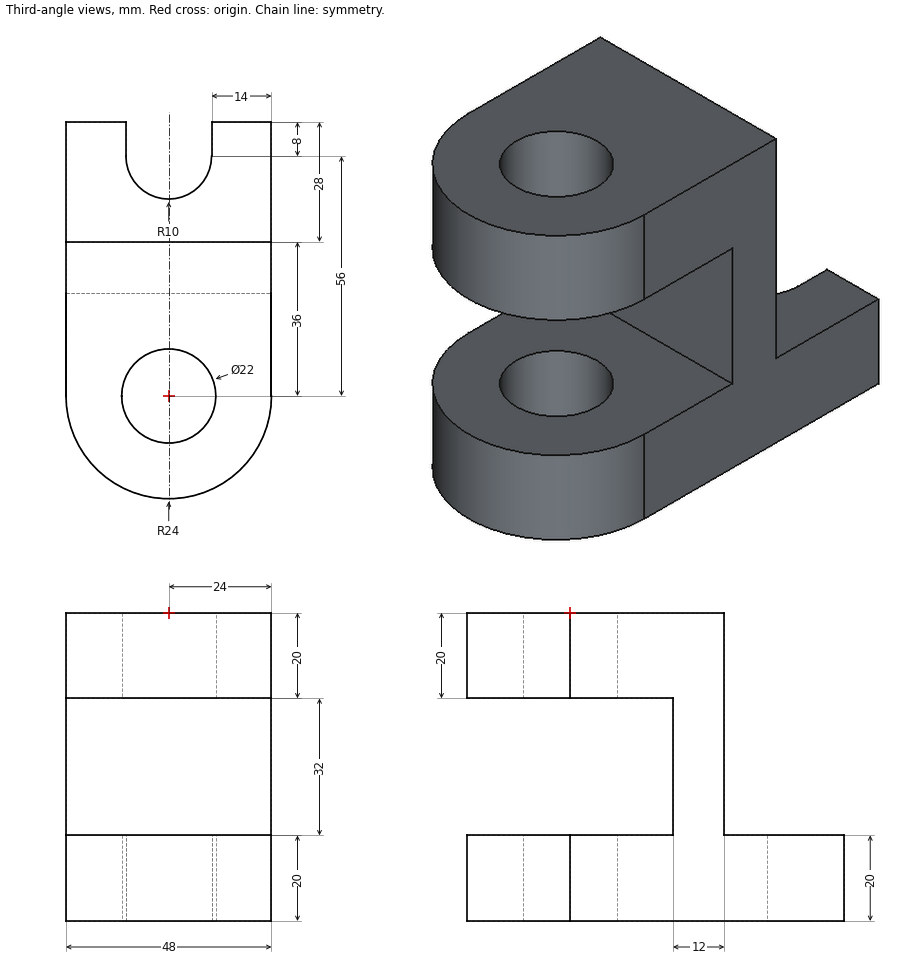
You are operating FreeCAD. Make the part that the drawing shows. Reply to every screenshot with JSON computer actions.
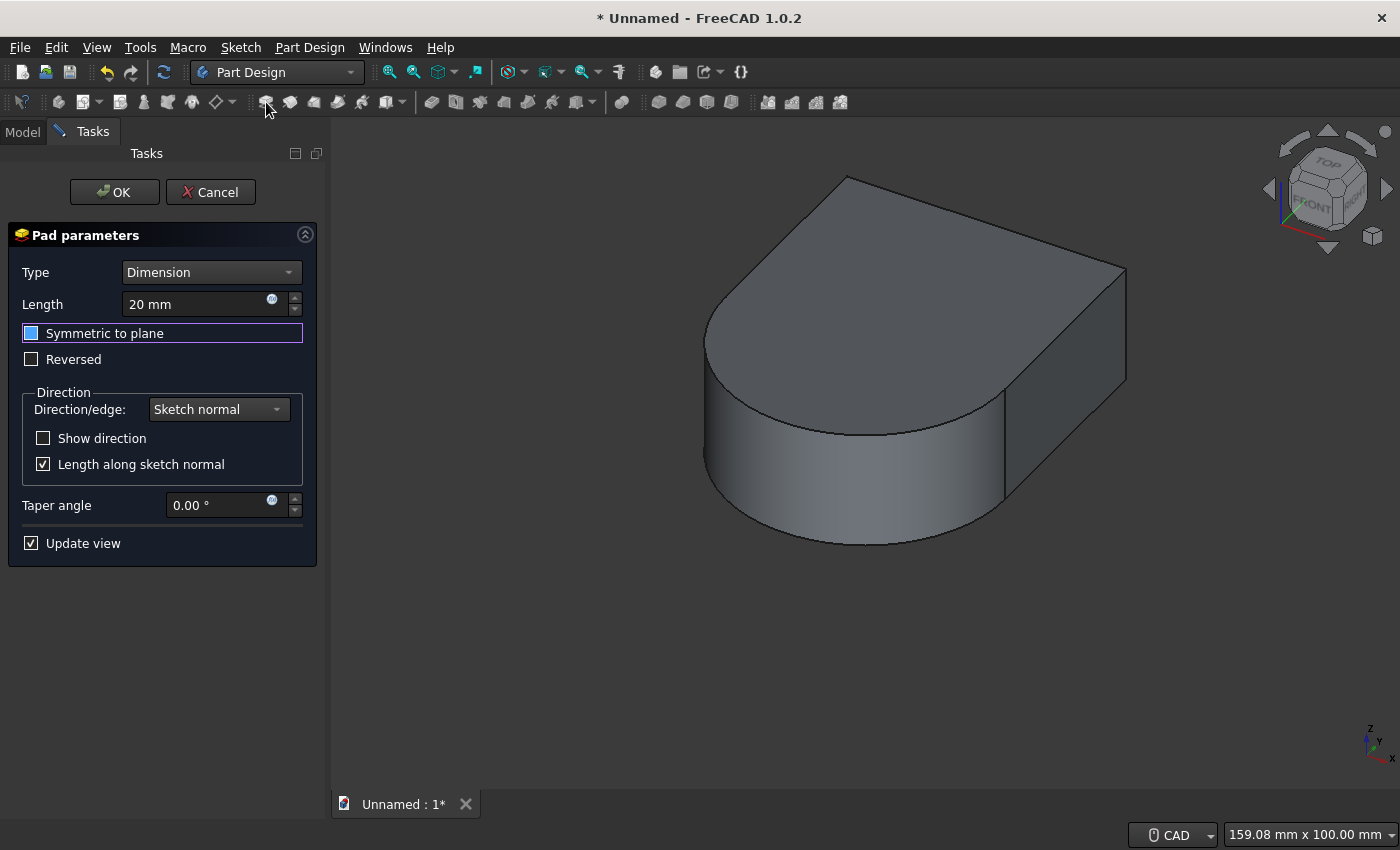
{"action": "left_click", "coordinate": [30, 359]}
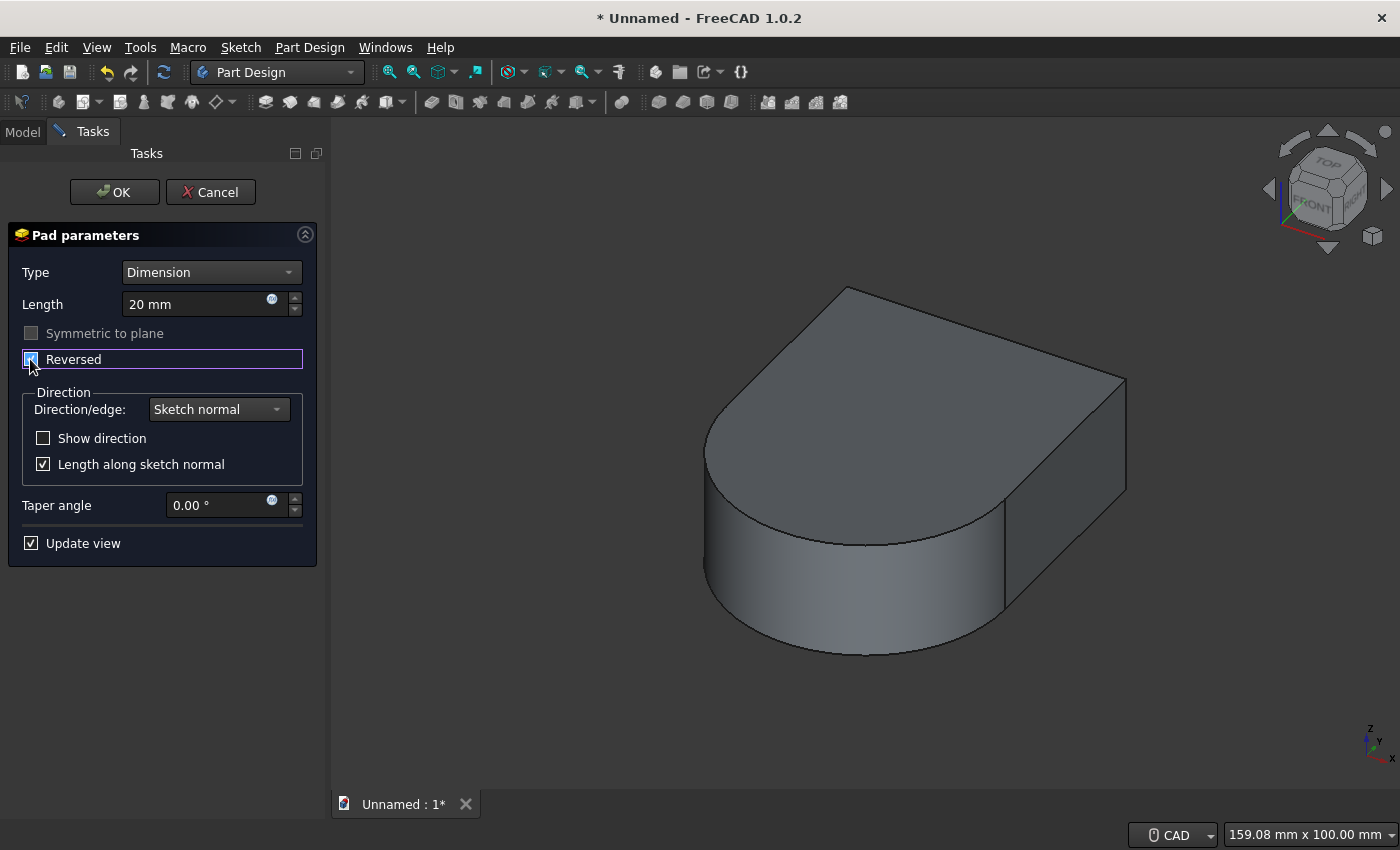
{"action": "left_click", "coordinate": [115, 192]}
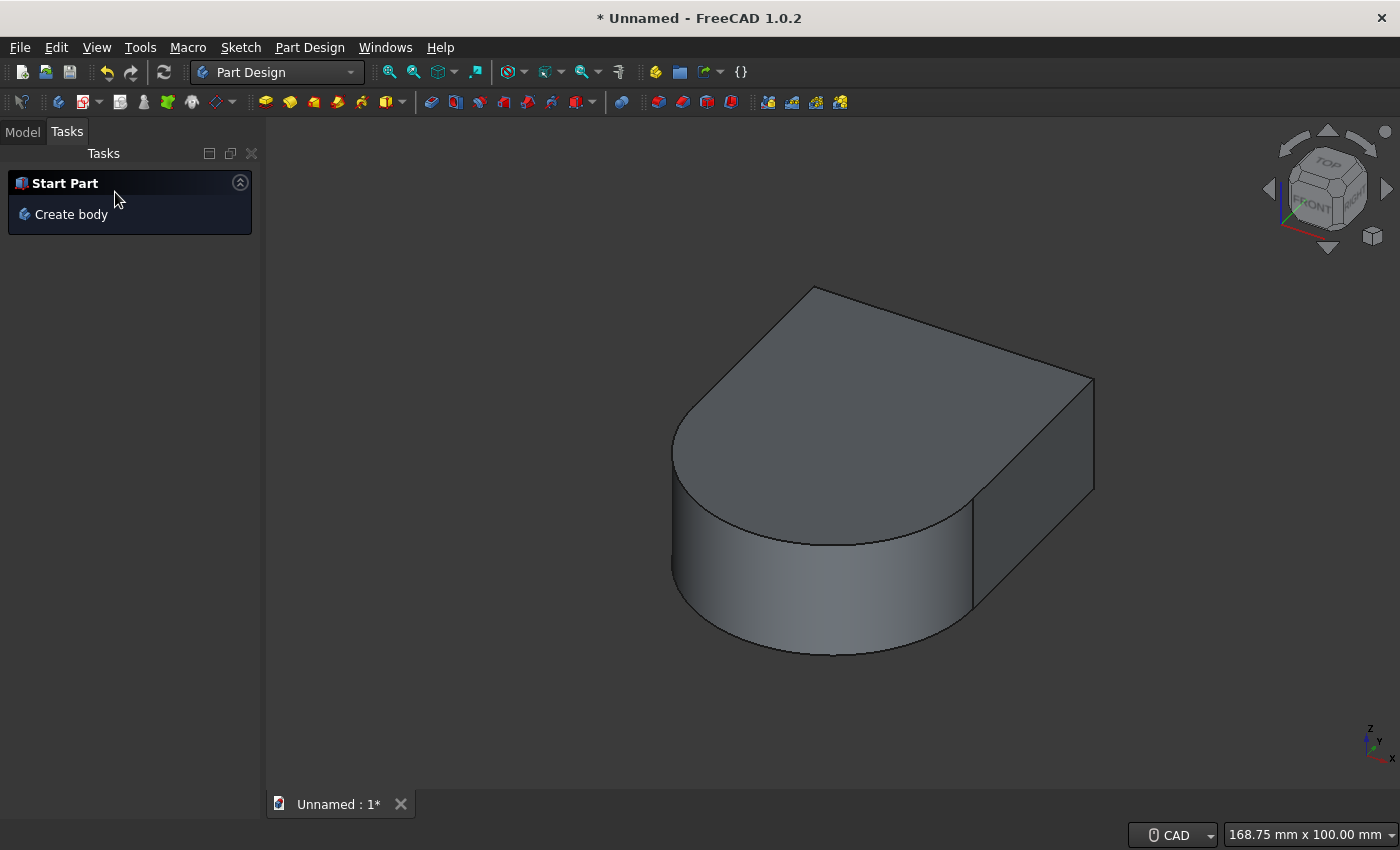
{"action": "left_click", "coordinate": [60, 102]}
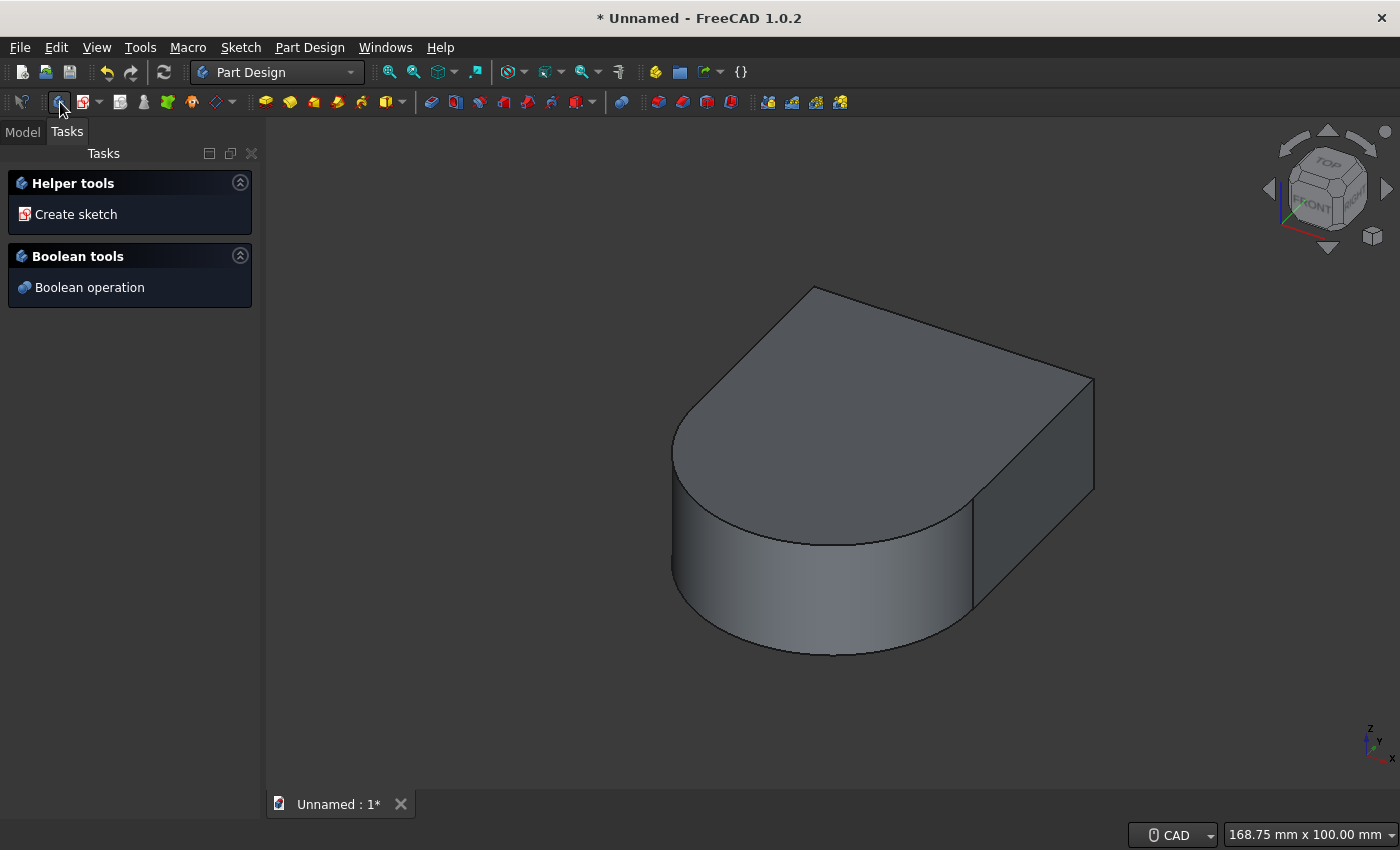
{"action": "left_click", "coordinate": [23, 131]}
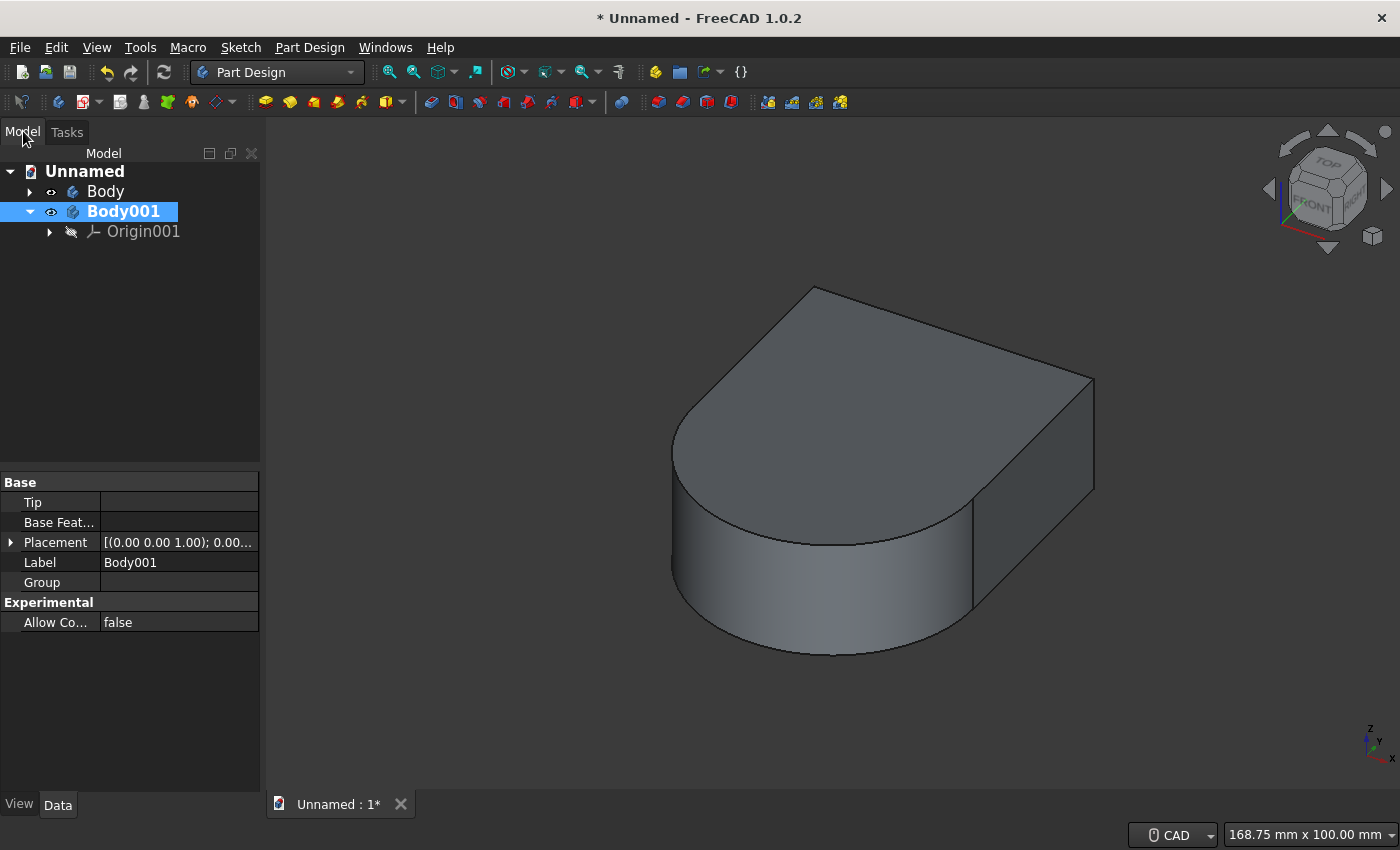
{"action": "left_click", "coordinate": [50, 232]}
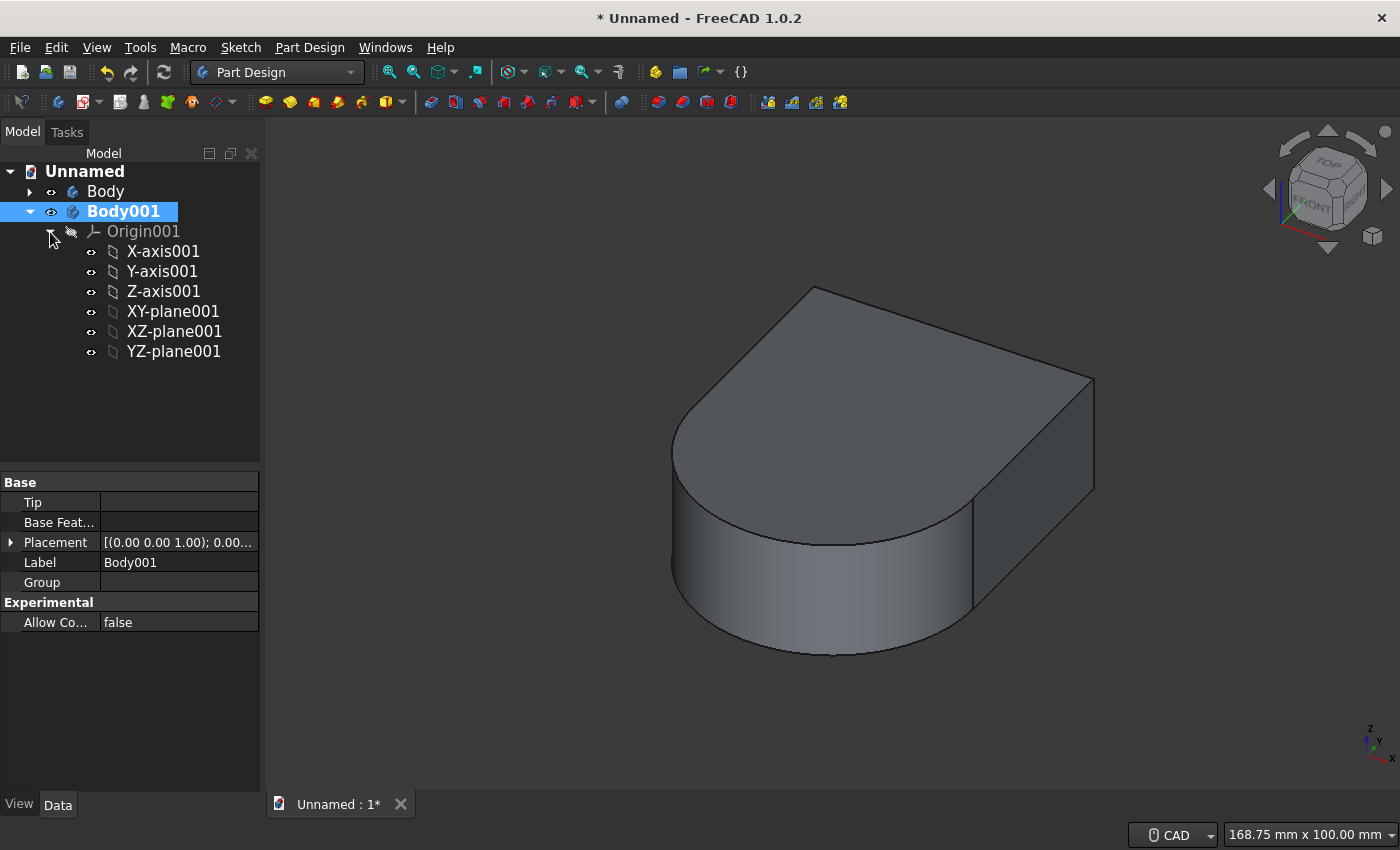
{"action": "left_click", "coordinate": [136, 312]}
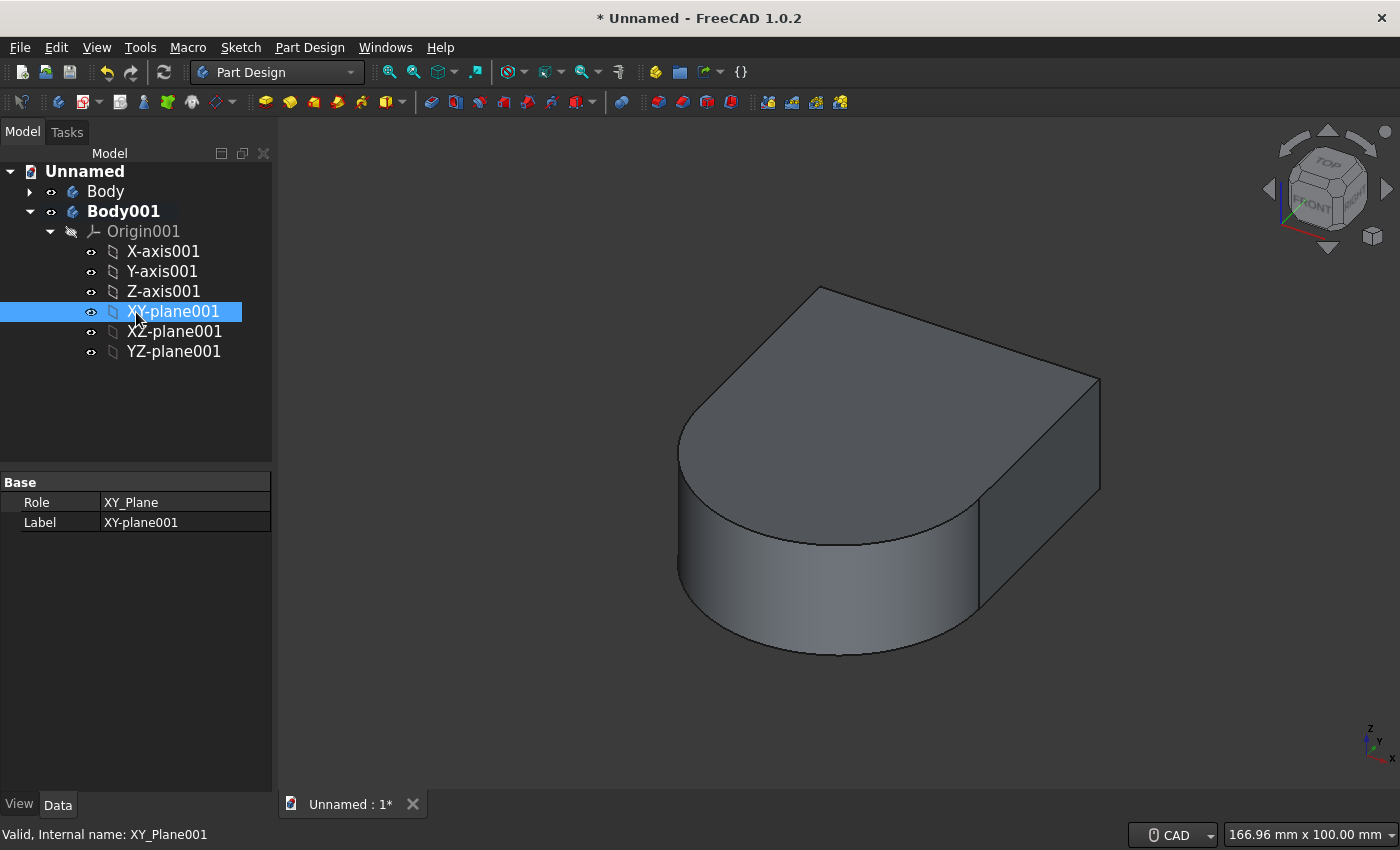
{"action": "left_click", "coordinate": [216, 102]}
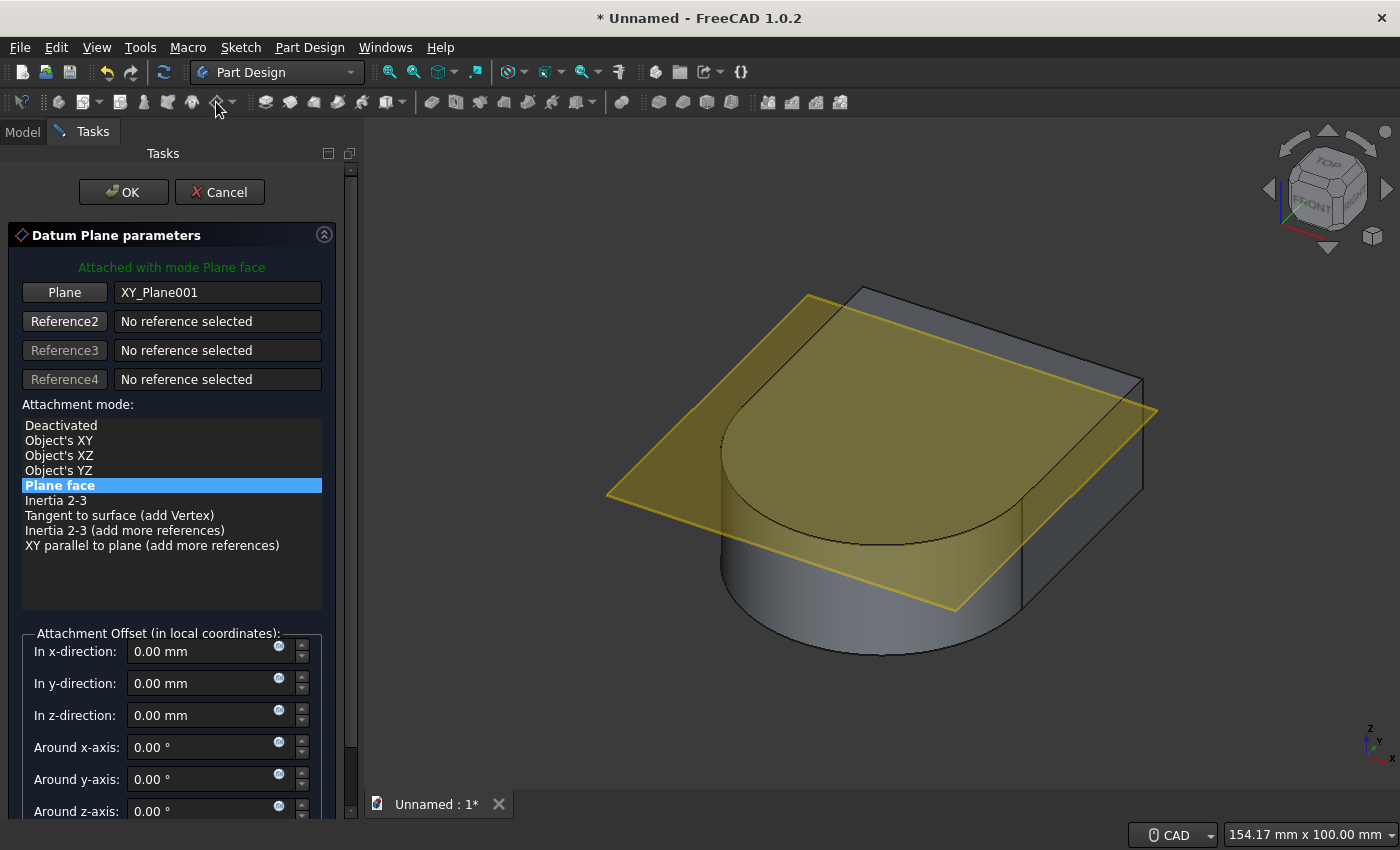
{"action": "triple_click", "coordinate": [210, 715]}